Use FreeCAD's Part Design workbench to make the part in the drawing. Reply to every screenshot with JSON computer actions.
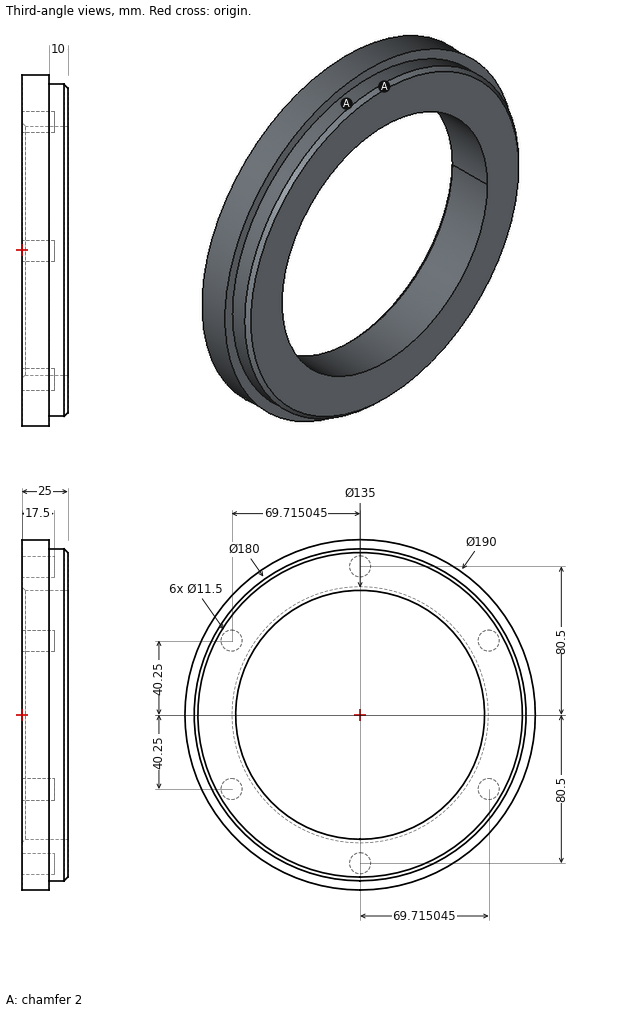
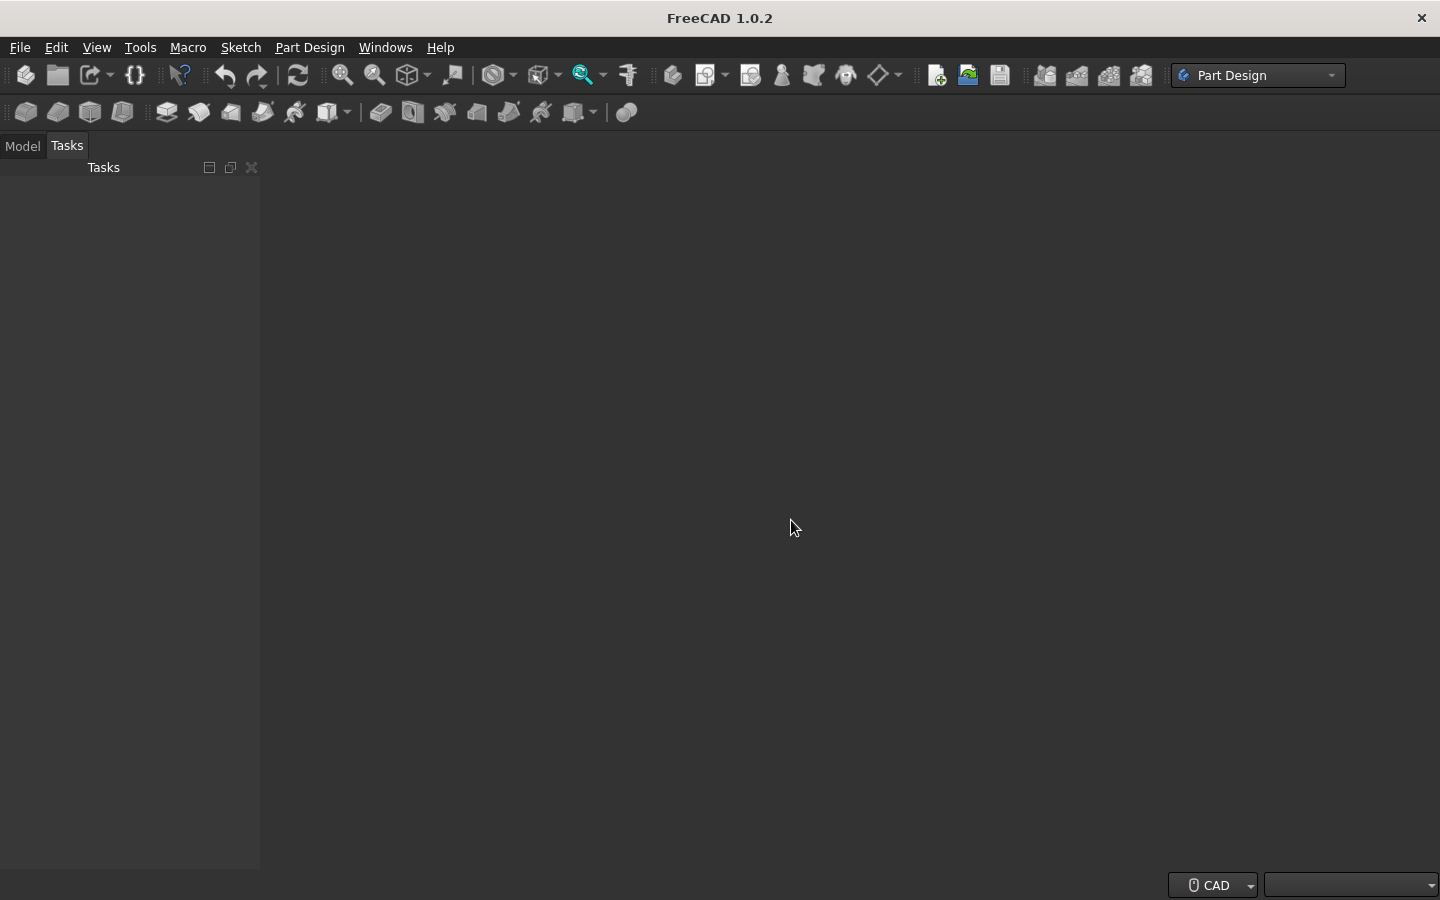
{"action": "left_click", "coordinate": [936, 76]}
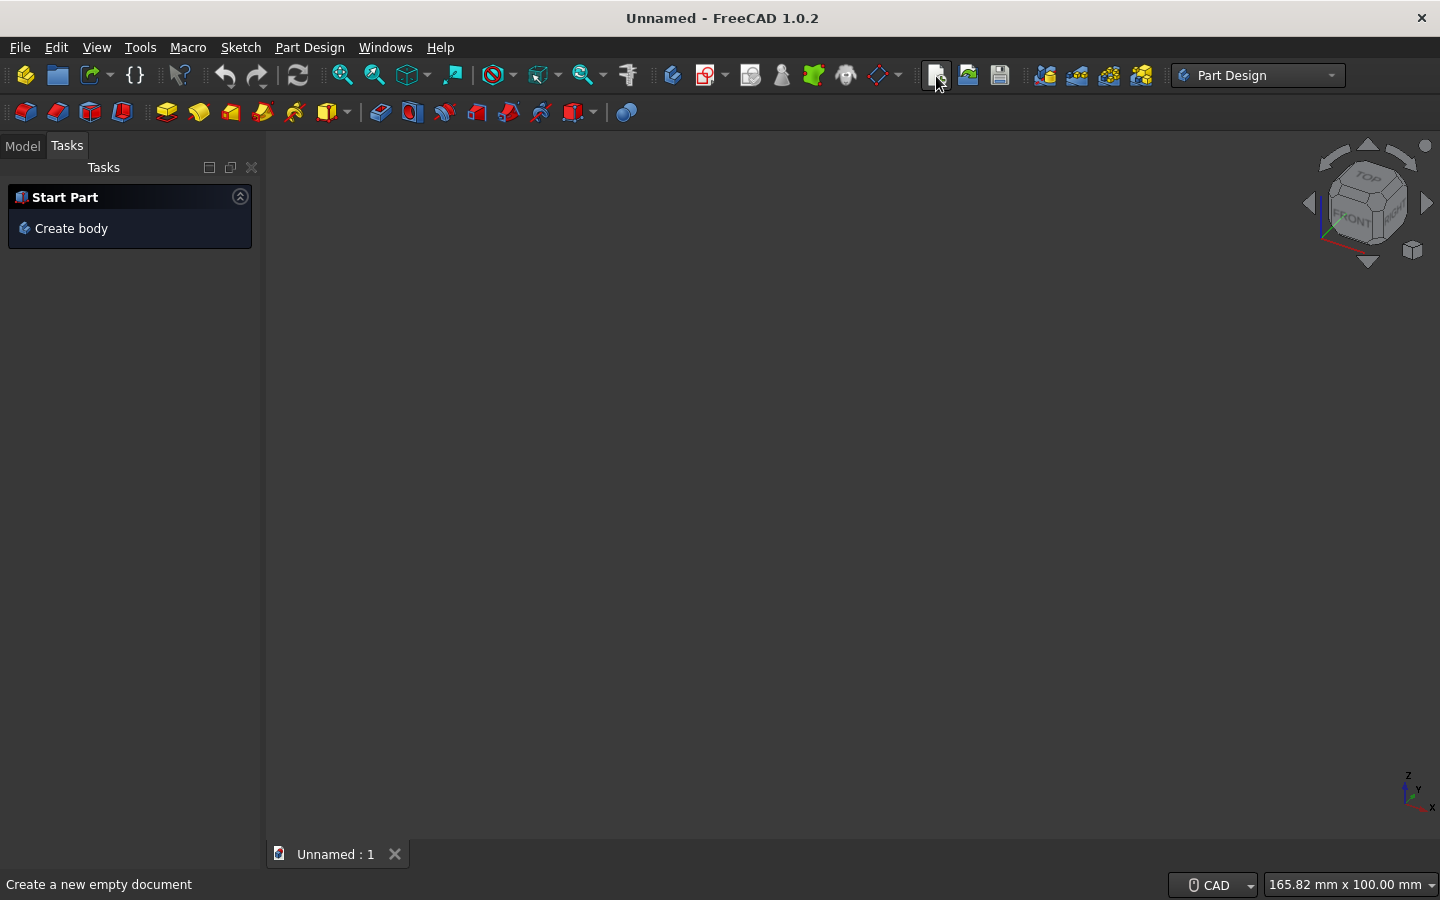
{"action": "left_click", "coordinate": [706, 76]}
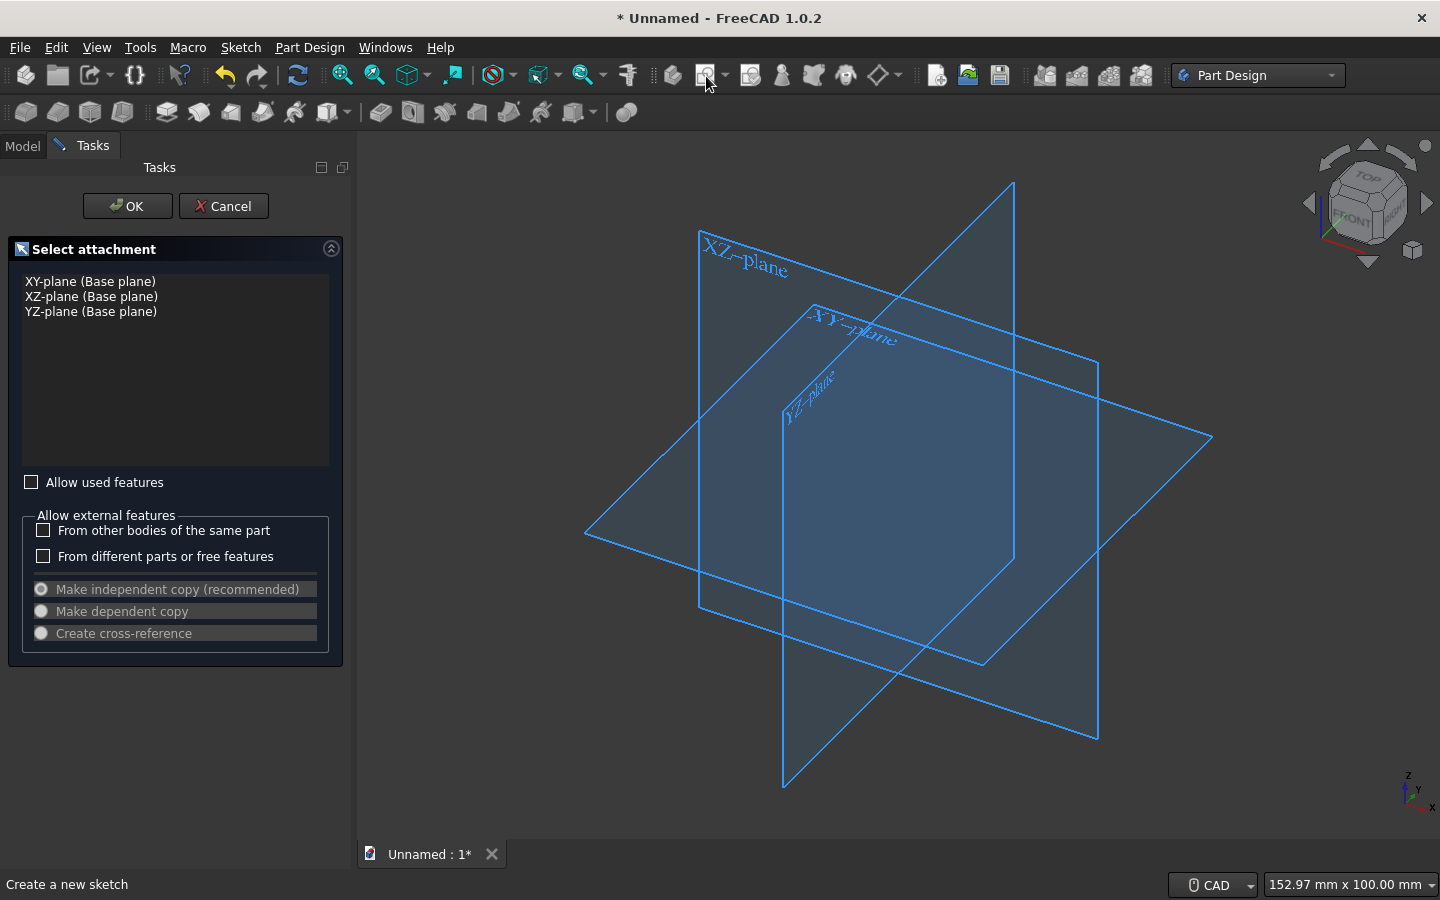
{"action": "left_click", "coordinate": [82, 312]}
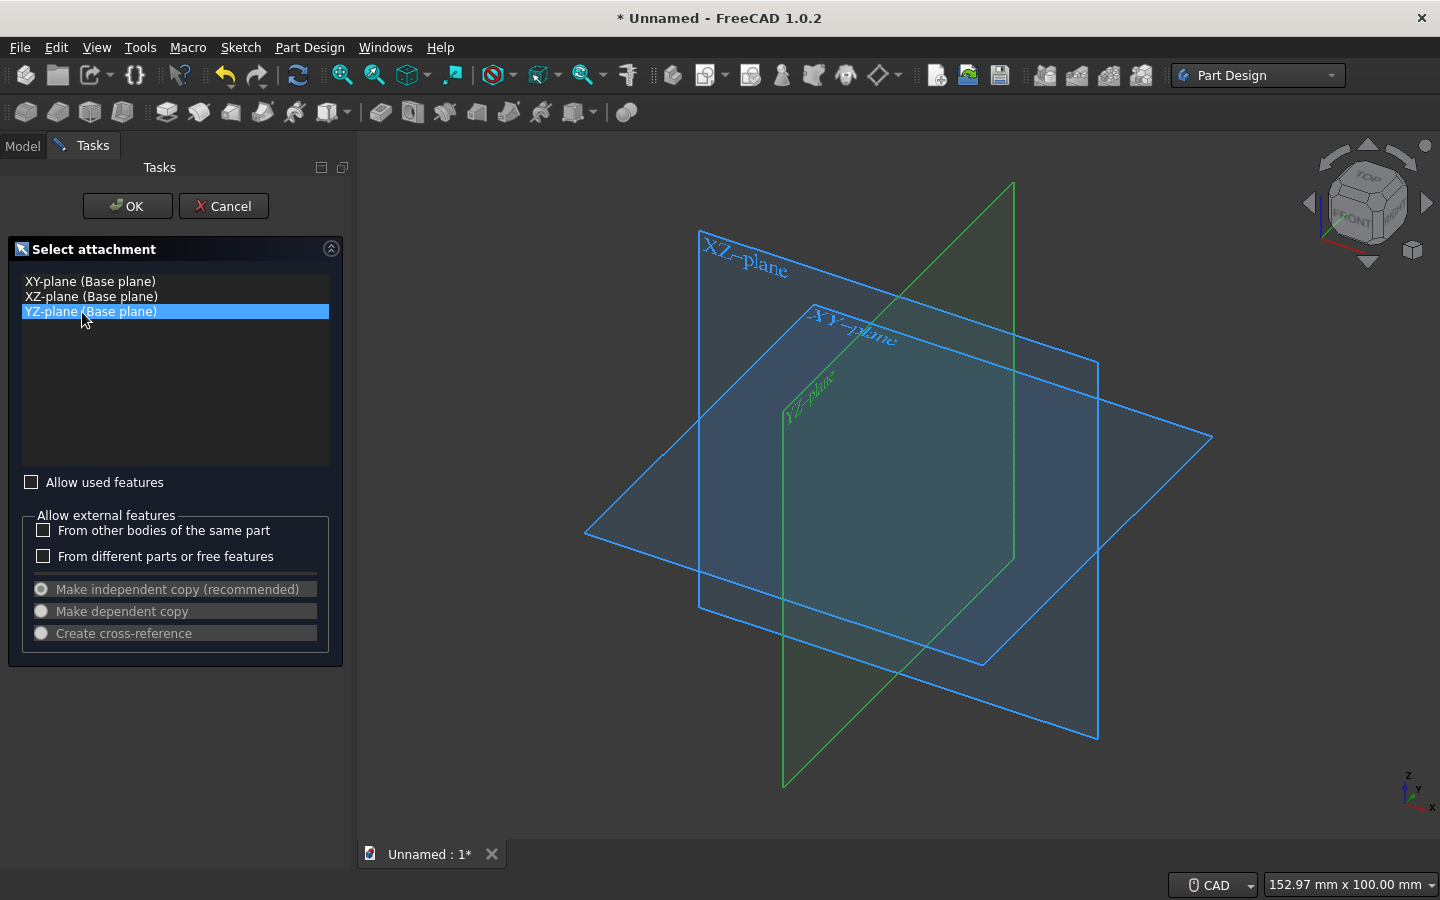
{"action": "left_click", "coordinate": [128, 206]}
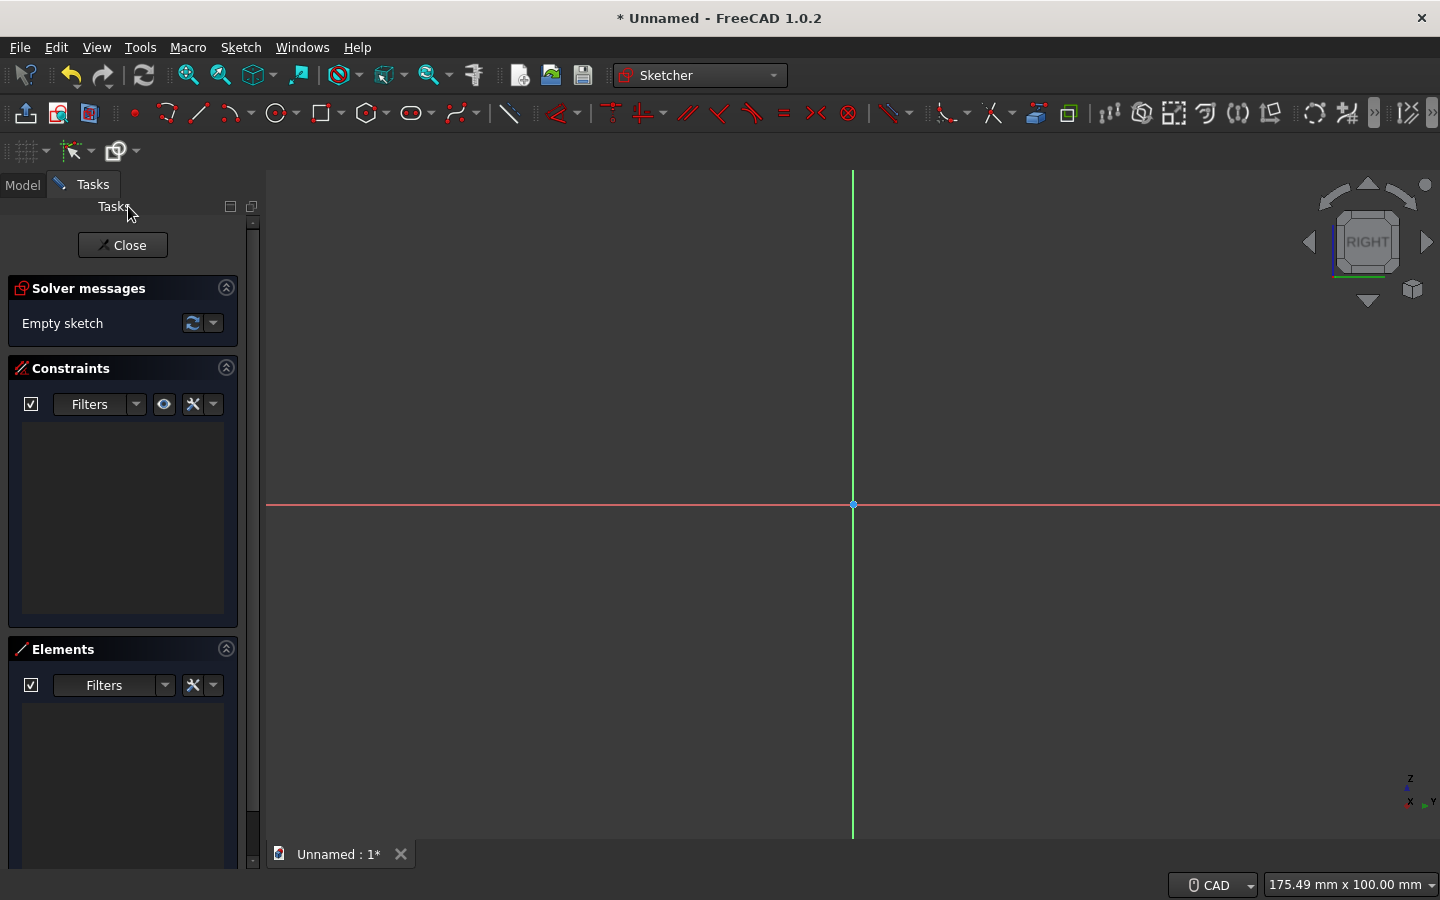
{"action": "scroll", "coordinate": [745, 504], "scroll_direction": "down", "scroll_amount": 5}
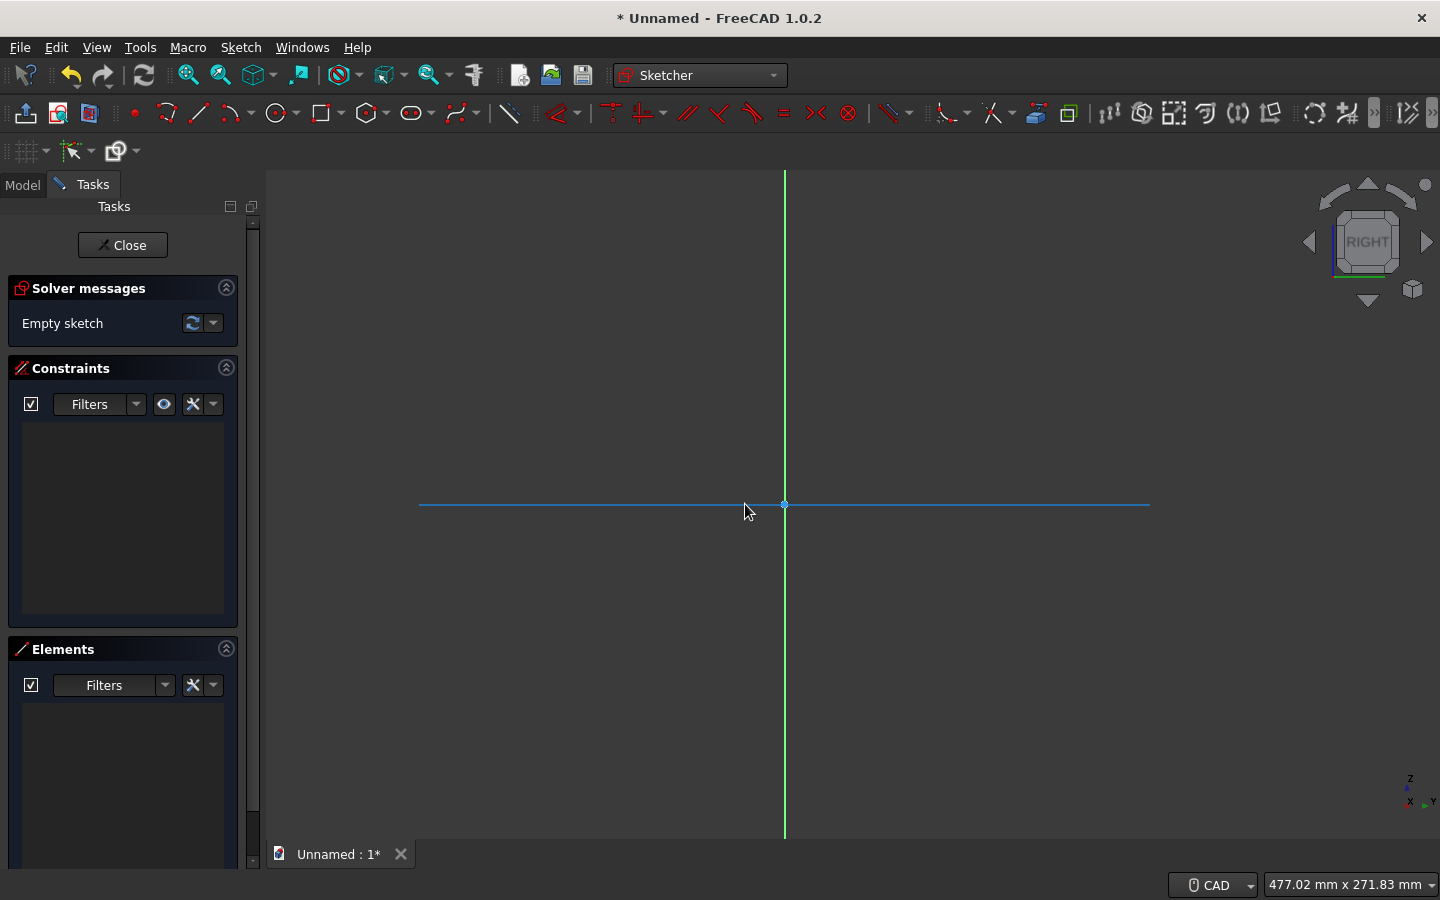
{"action": "left_click", "coordinate": [276, 114]}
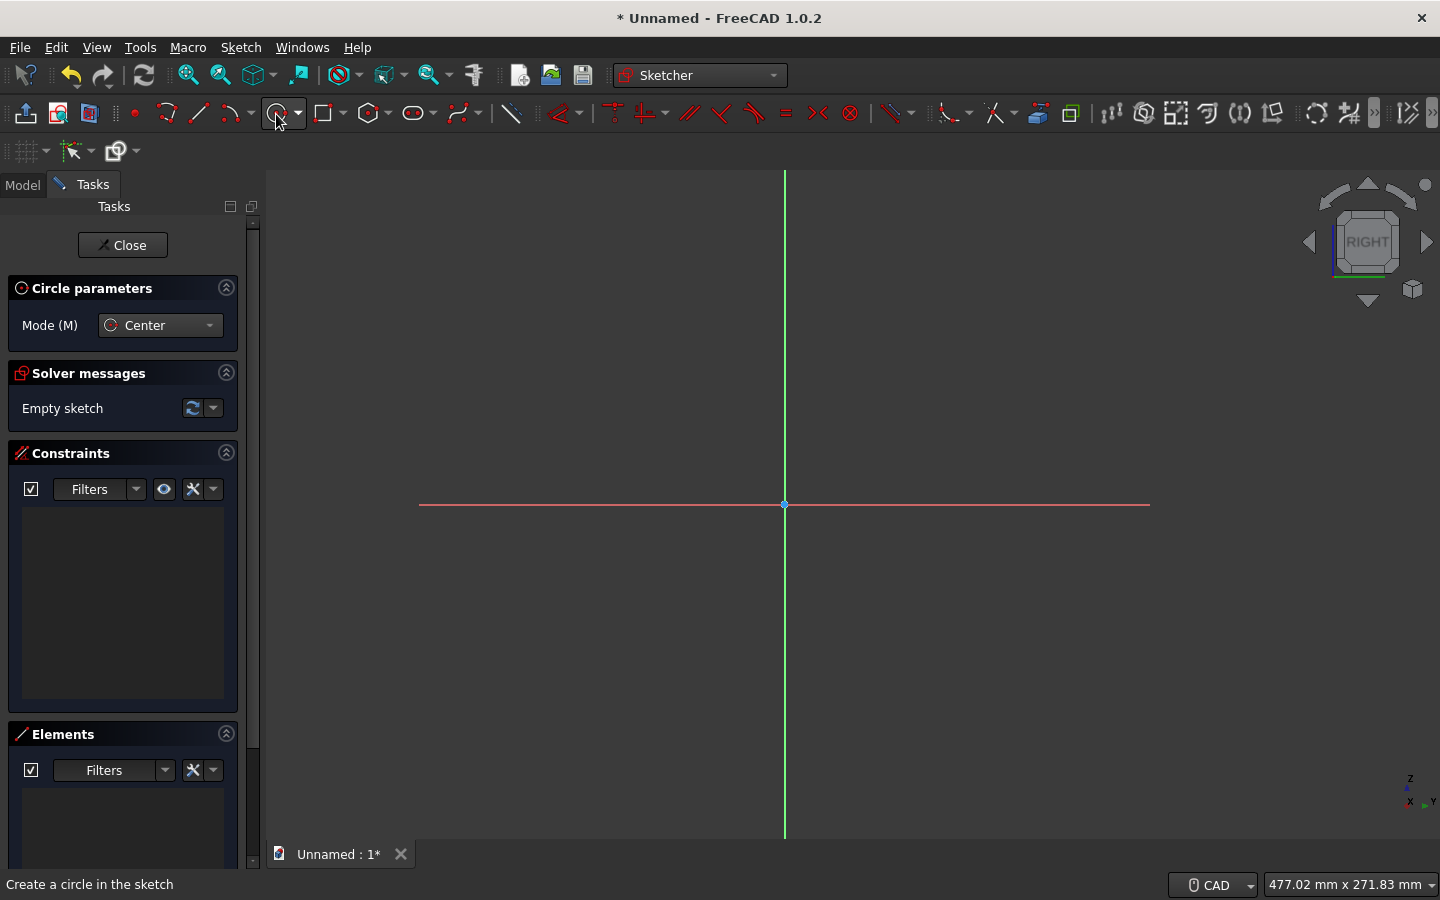
{"action": "left_click", "coordinate": [785, 504]}
{"action": "left_click", "coordinate": [950, 339]}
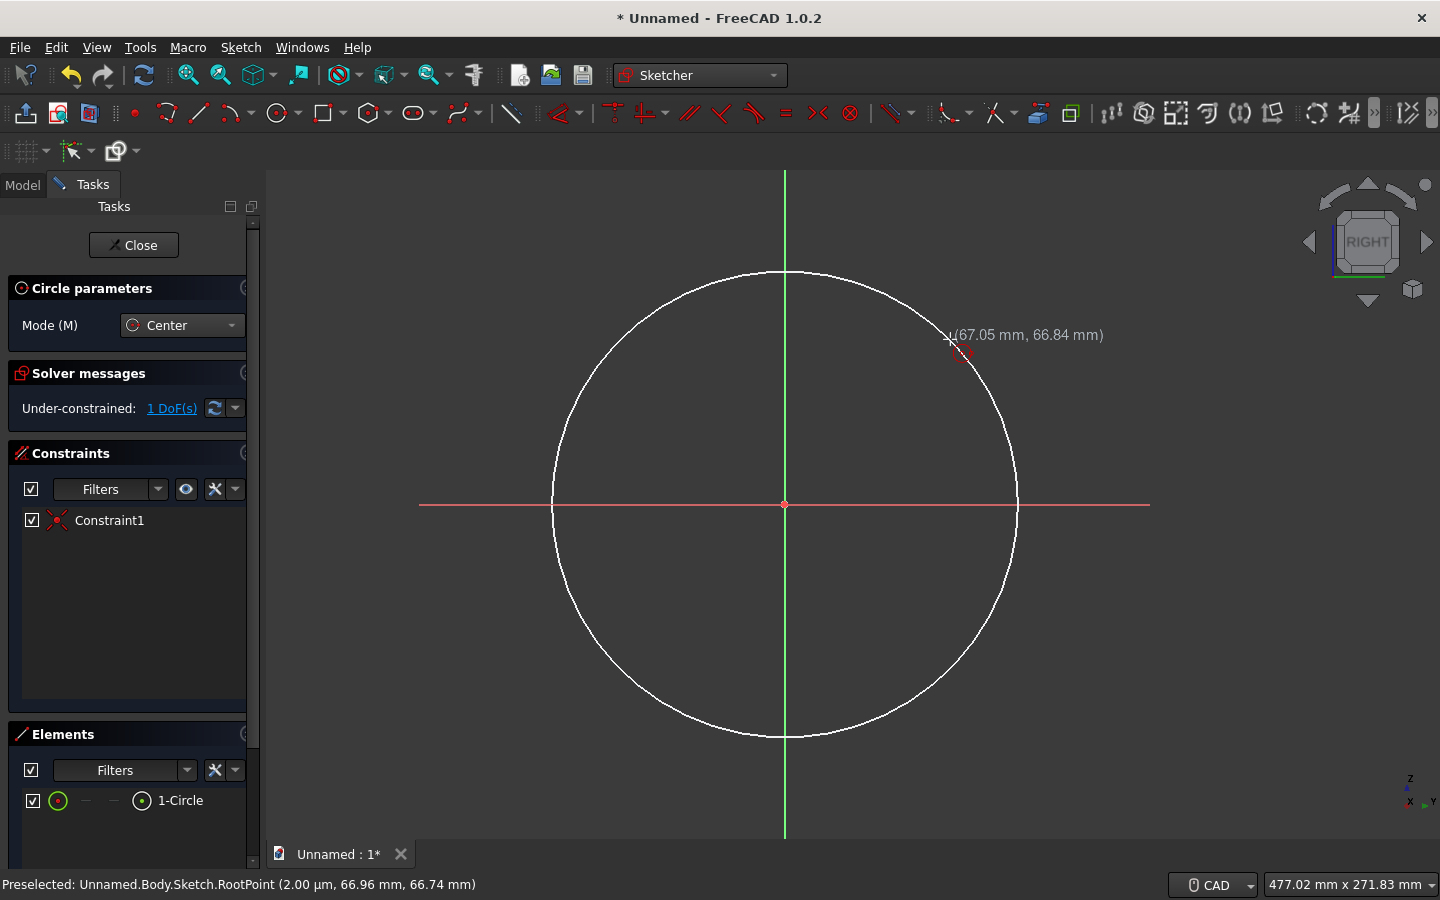
{"action": "left_click", "coordinate": [785, 504]}
{"action": "left_click", "coordinate": [902, 387]}
{"action": "key", "text": "Escape"}